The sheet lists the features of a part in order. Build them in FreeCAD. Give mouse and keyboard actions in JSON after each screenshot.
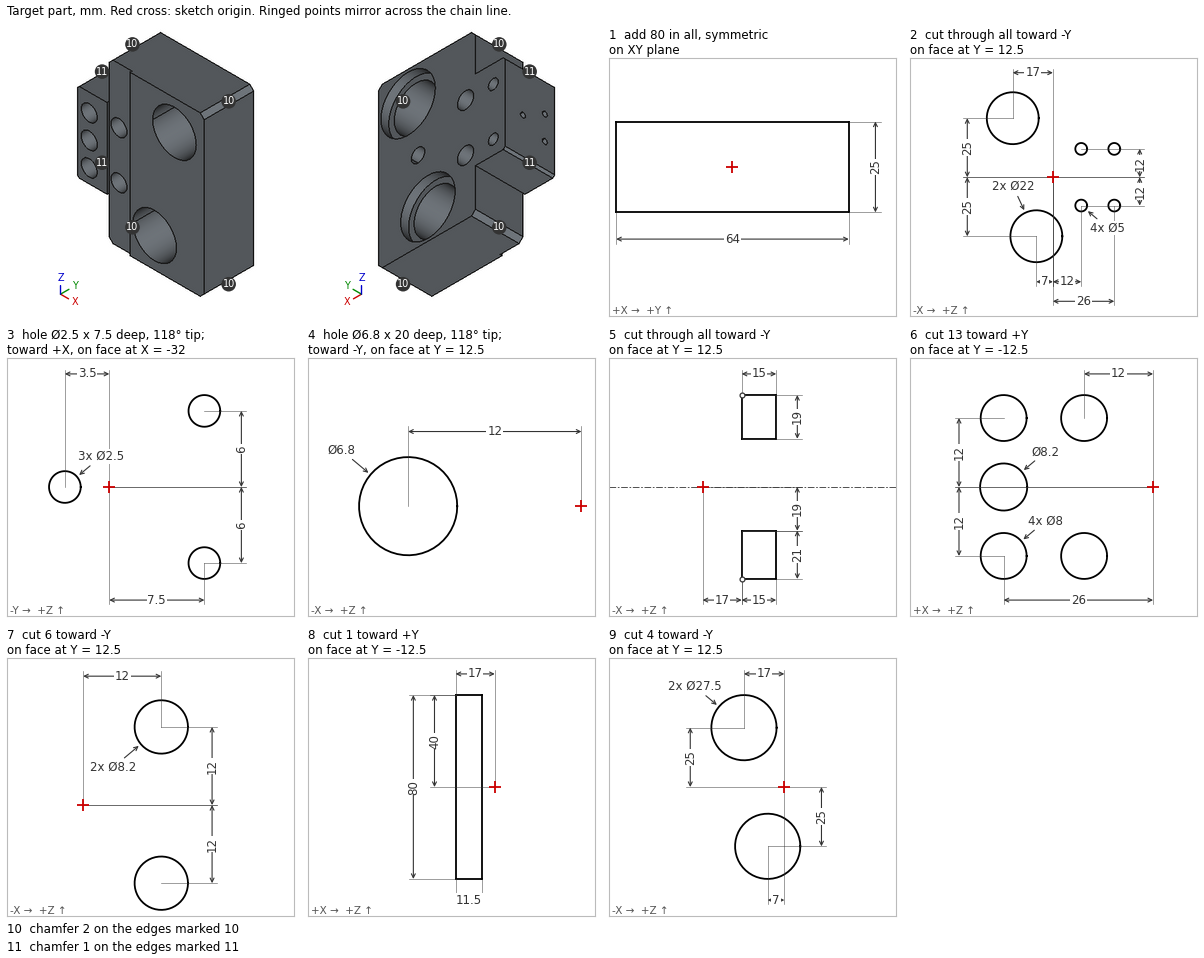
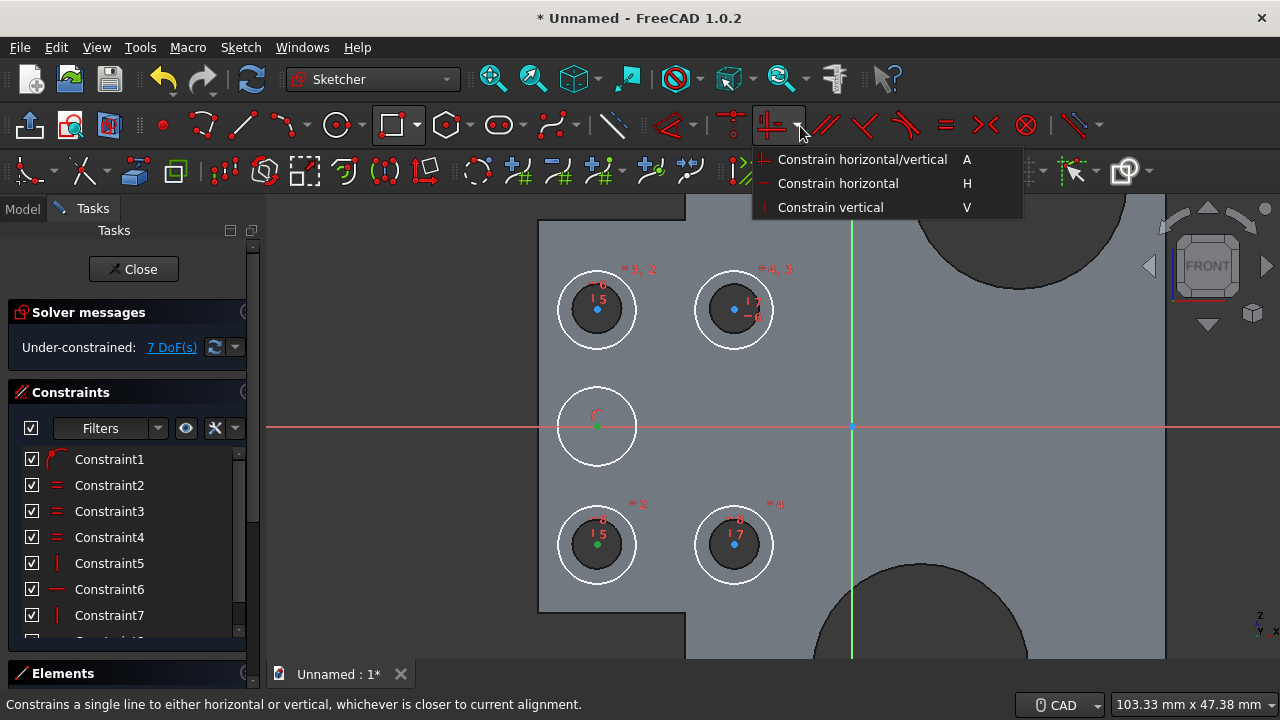
{"action": "left_click", "coordinate": [888, 207]}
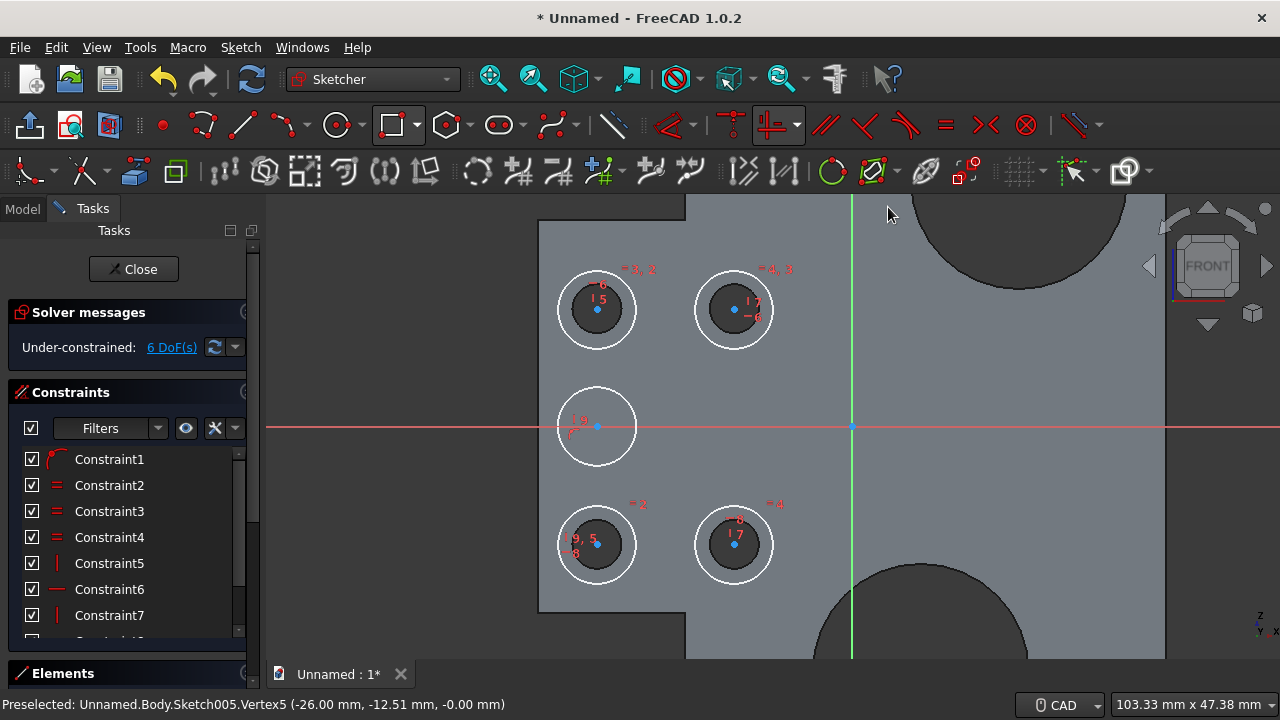
{"action": "left_click", "coordinate": [668, 126]}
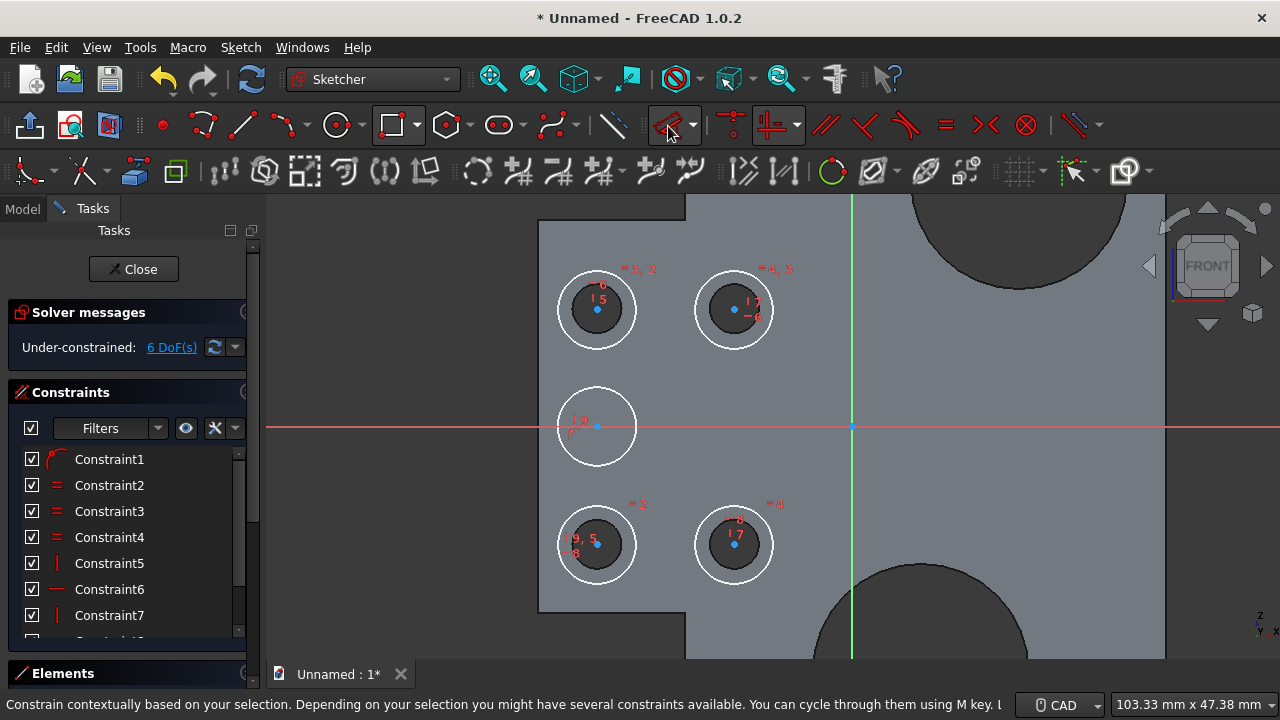
{"action": "left_click", "coordinate": [624, 517]}
{"action": "left_click", "coordinate": [646, 494]}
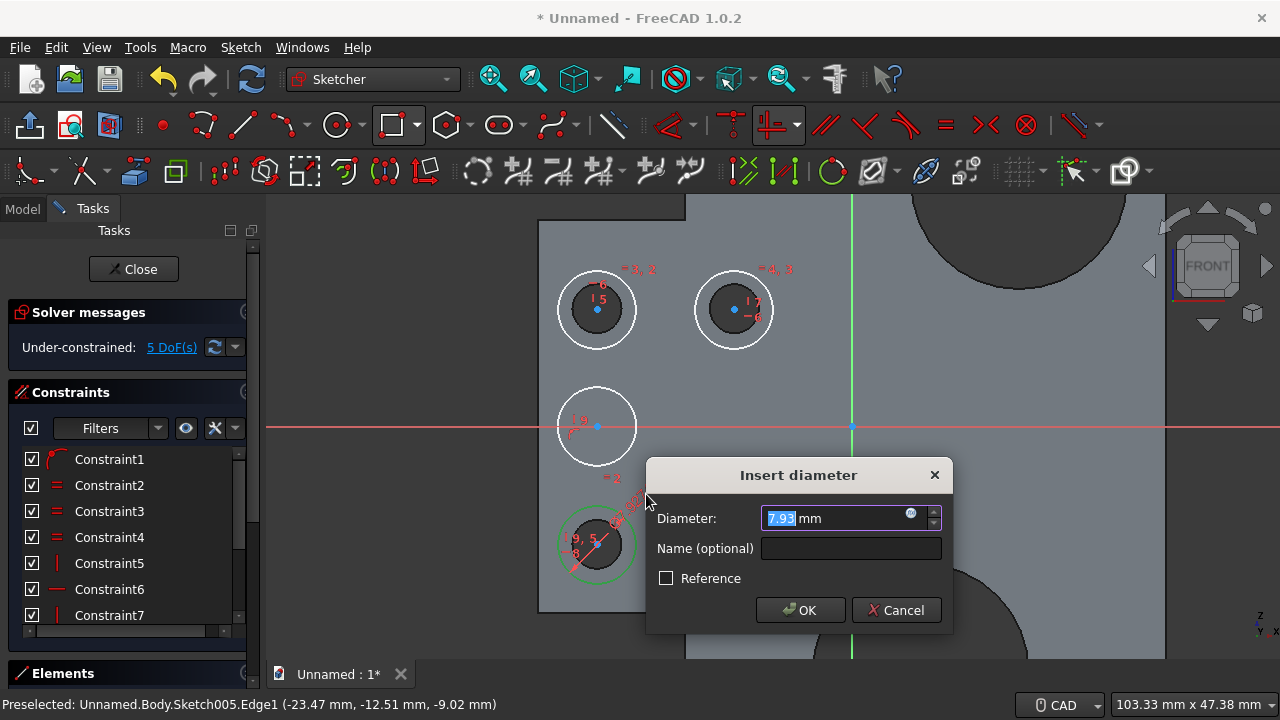
{"action": "type", "text": "8"}
{"action": "key", "text": "Return"}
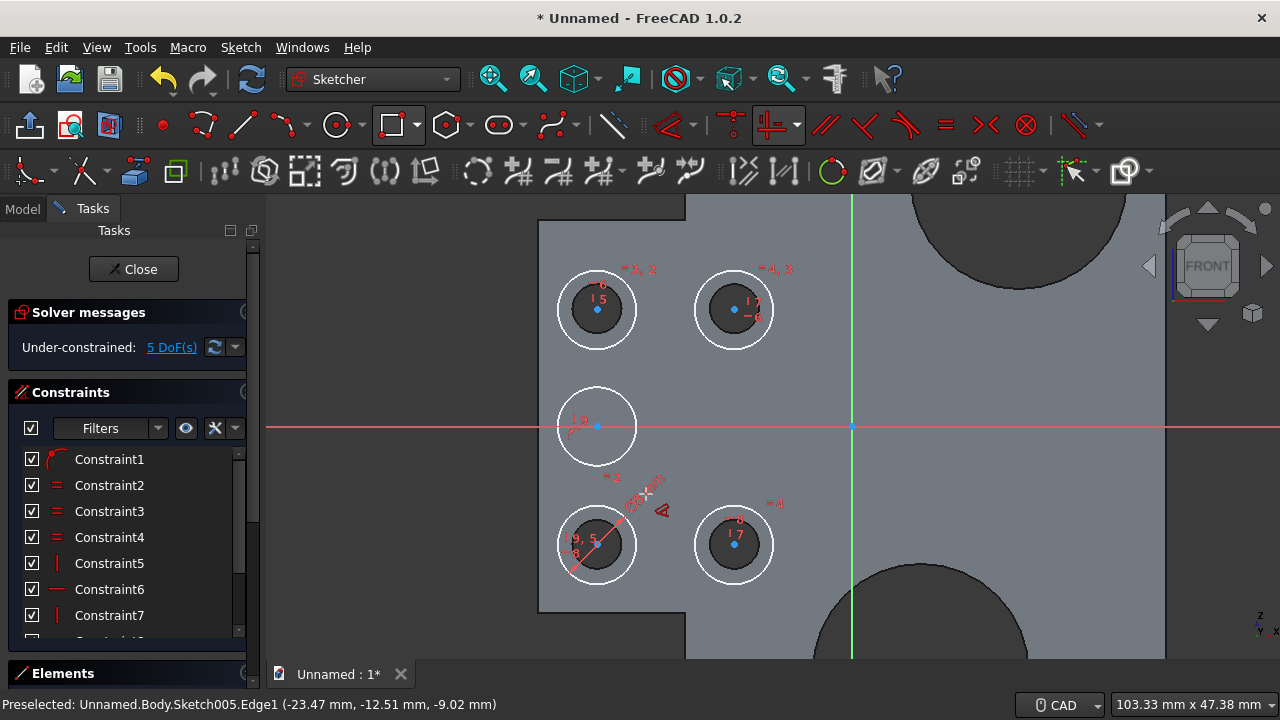
{"action": "left_click", "coordinate": [625, 399]}
{"action": "left_click", "coordinate": [648, 377]}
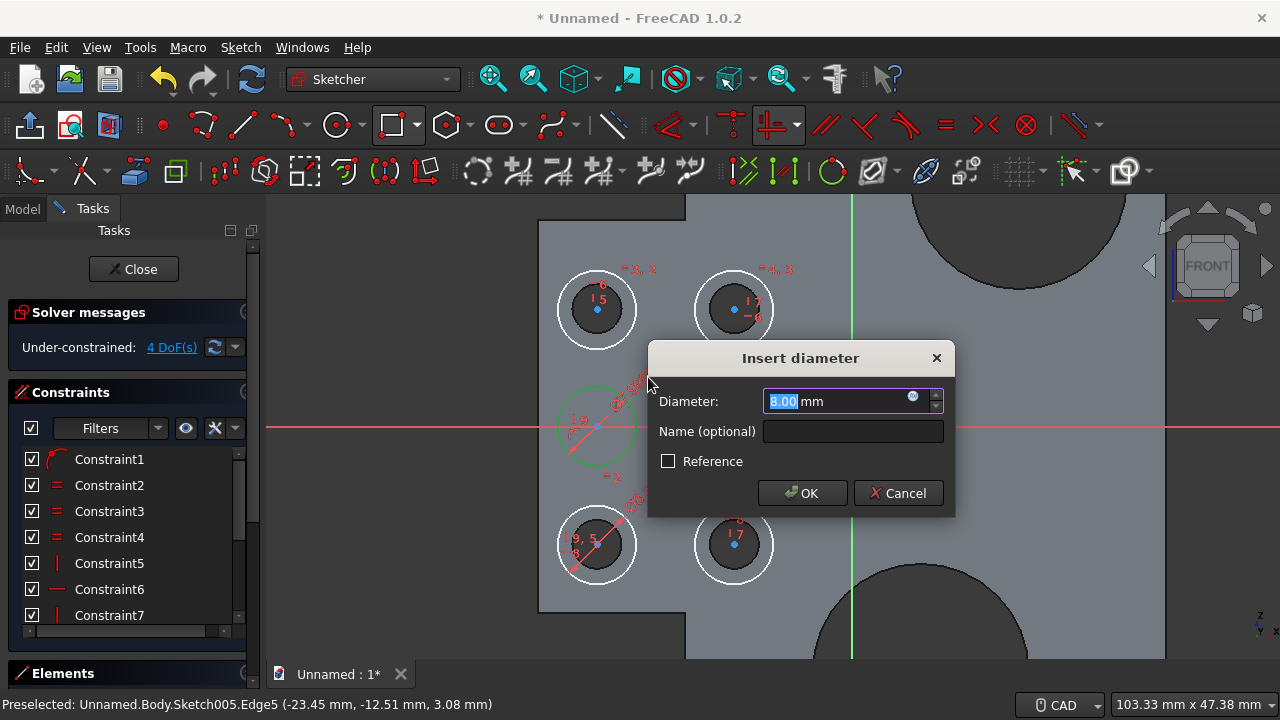
{"action": "type", "text": "8.2"}
{"action": "key", "text": "Return"}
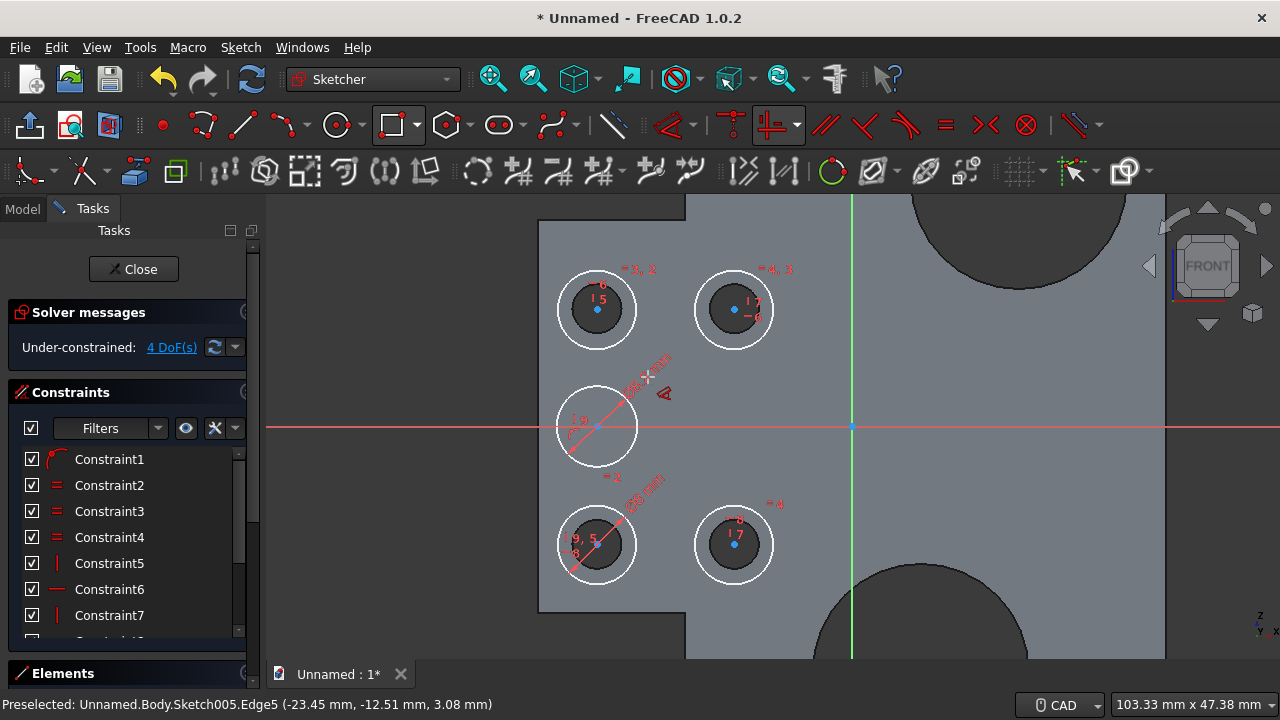
{"action": "left_click", "coordinate": [597, 545]}
{"action": "left_click", "coordinate": [666, 579]}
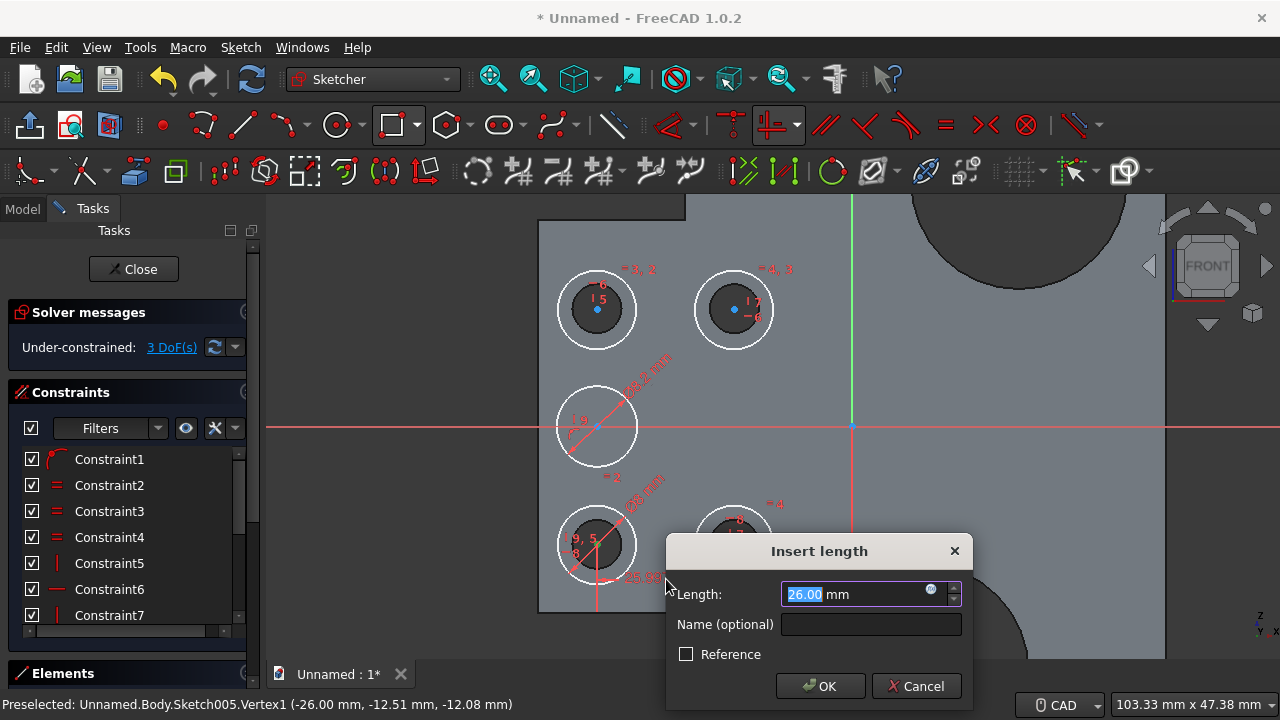
{"action": "type", "text": "26"}
{"action": "key", "text": "Return"}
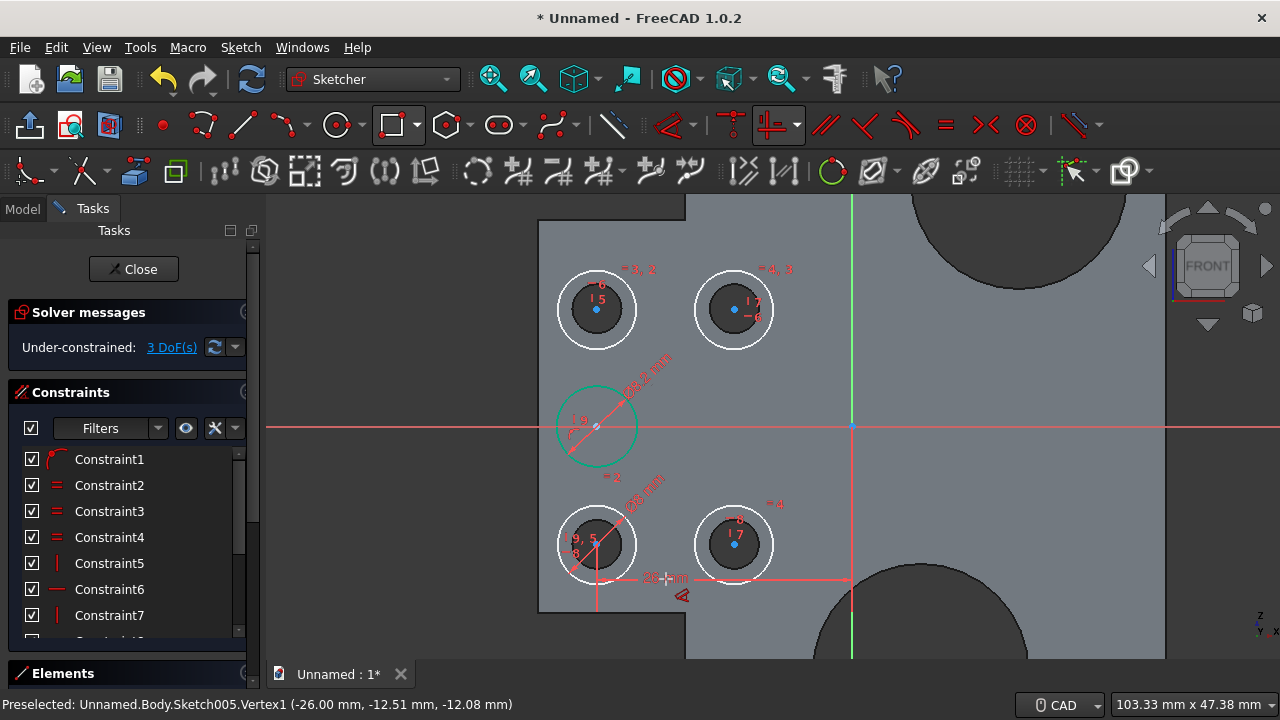
{"action": "left_click", "coordinate": [597, 545]}
{"action": "left_click", "coordinate": [886, 486]}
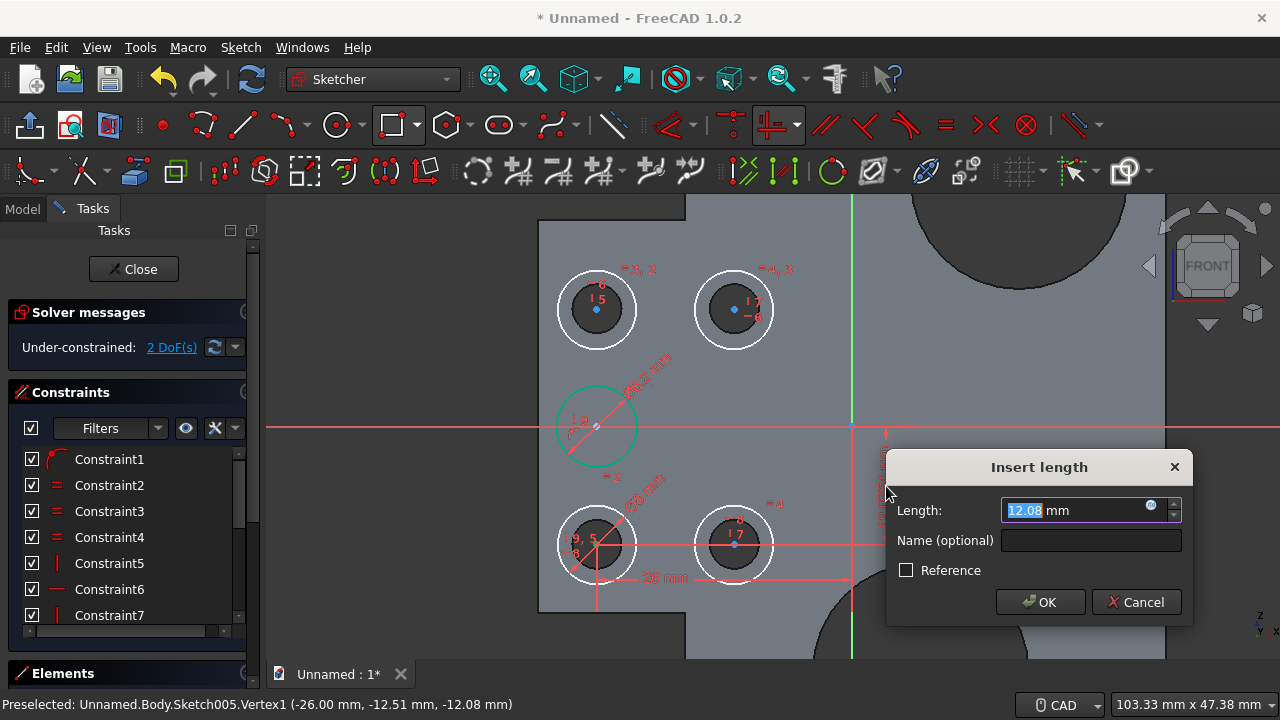
{"action": "type", "text": "12"}
{"action": "key", "text": "Return"}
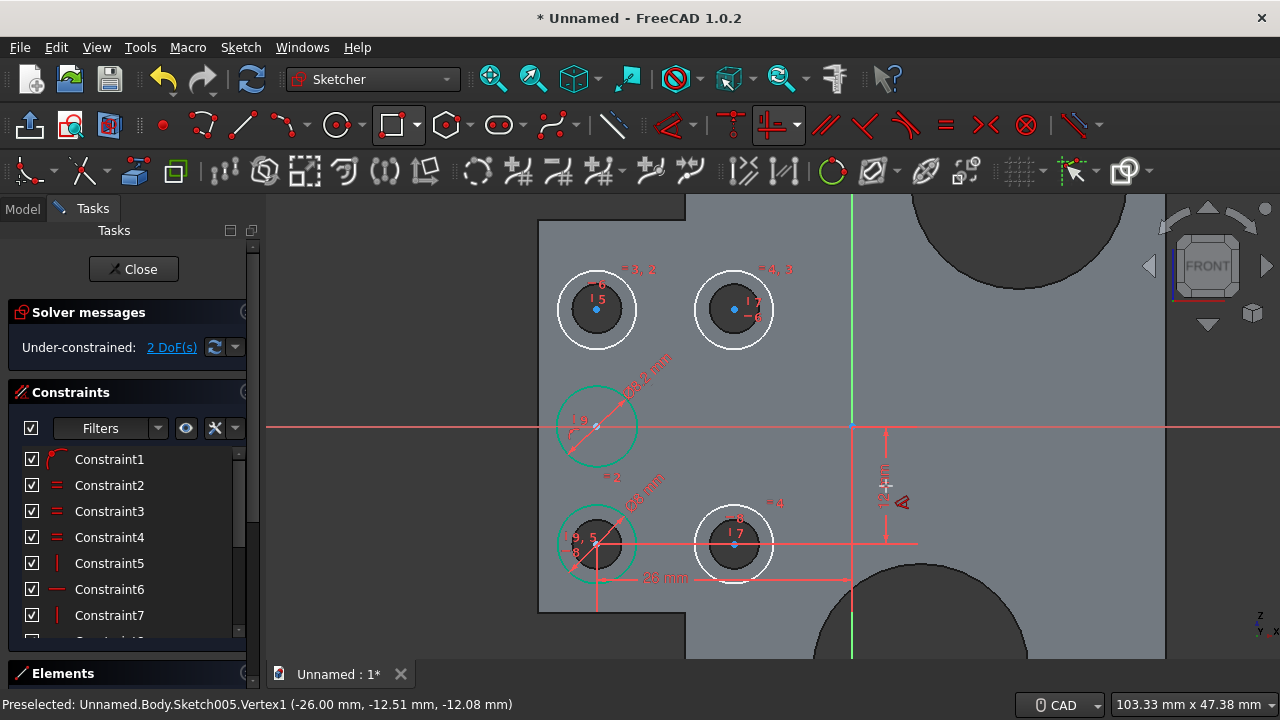
{"action": "left_click", "coordinate": [597, 310]}
{"action": "left_click", "coordinate": [886, 368]}